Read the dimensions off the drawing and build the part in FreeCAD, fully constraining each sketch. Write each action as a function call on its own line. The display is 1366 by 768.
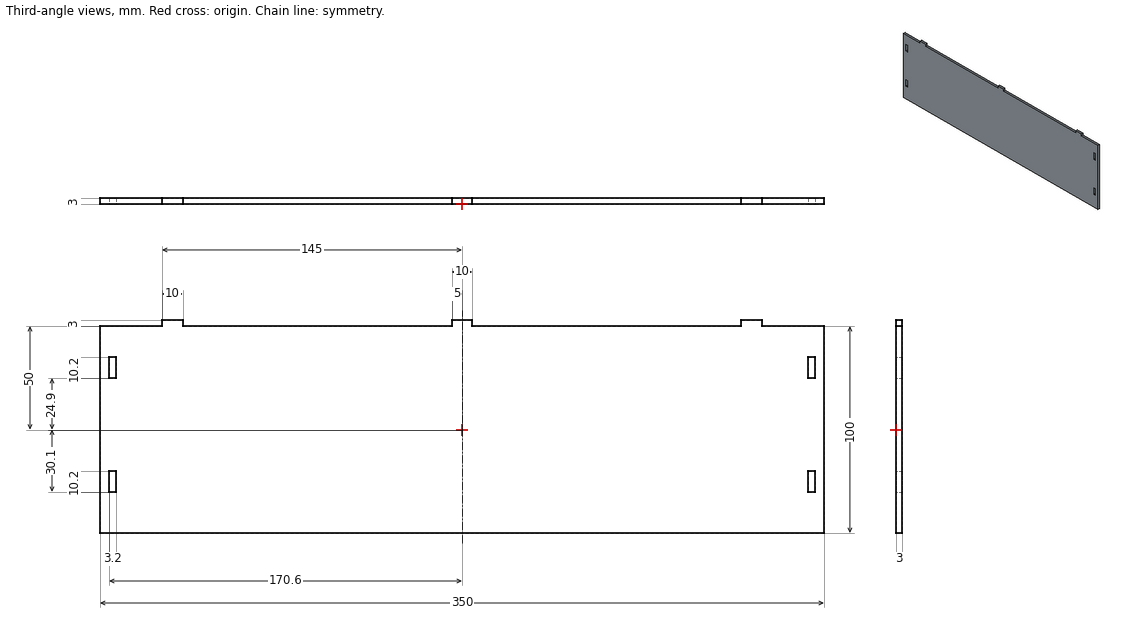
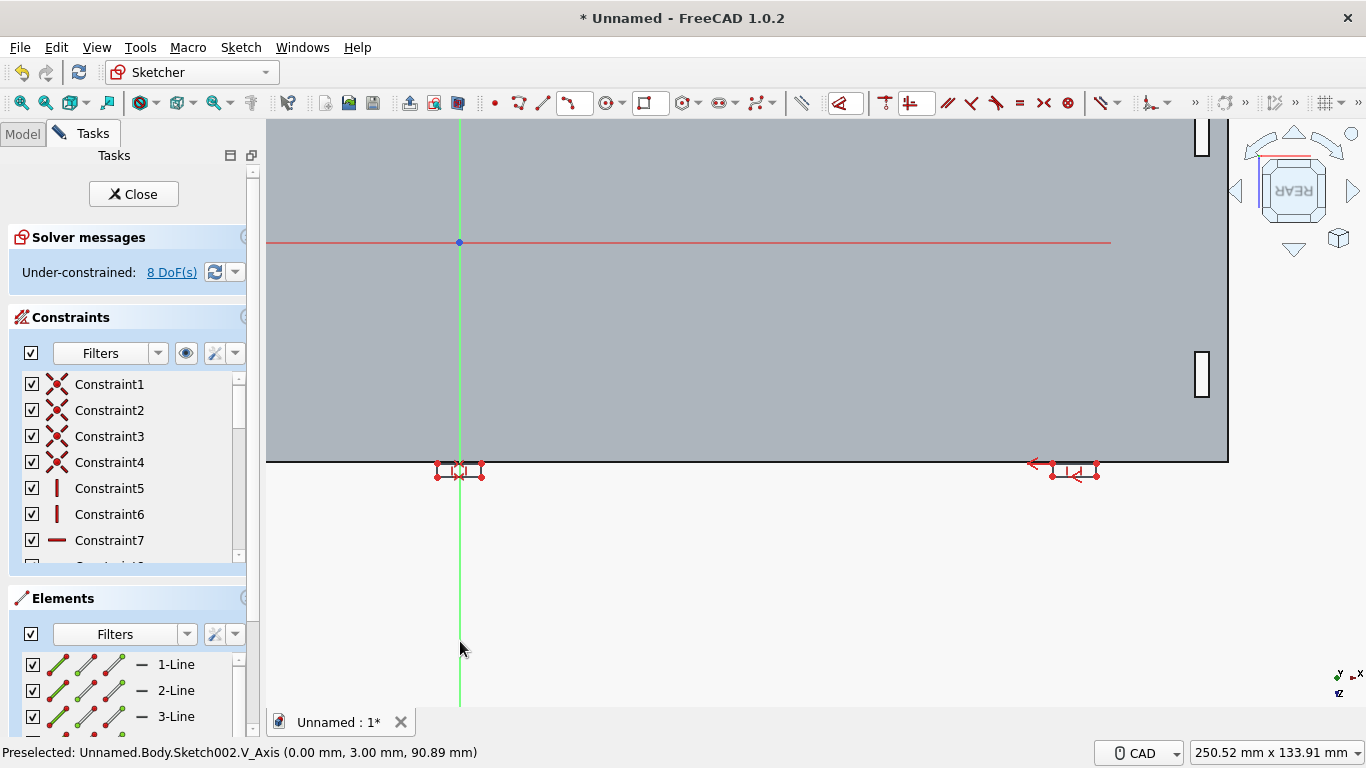
key(d)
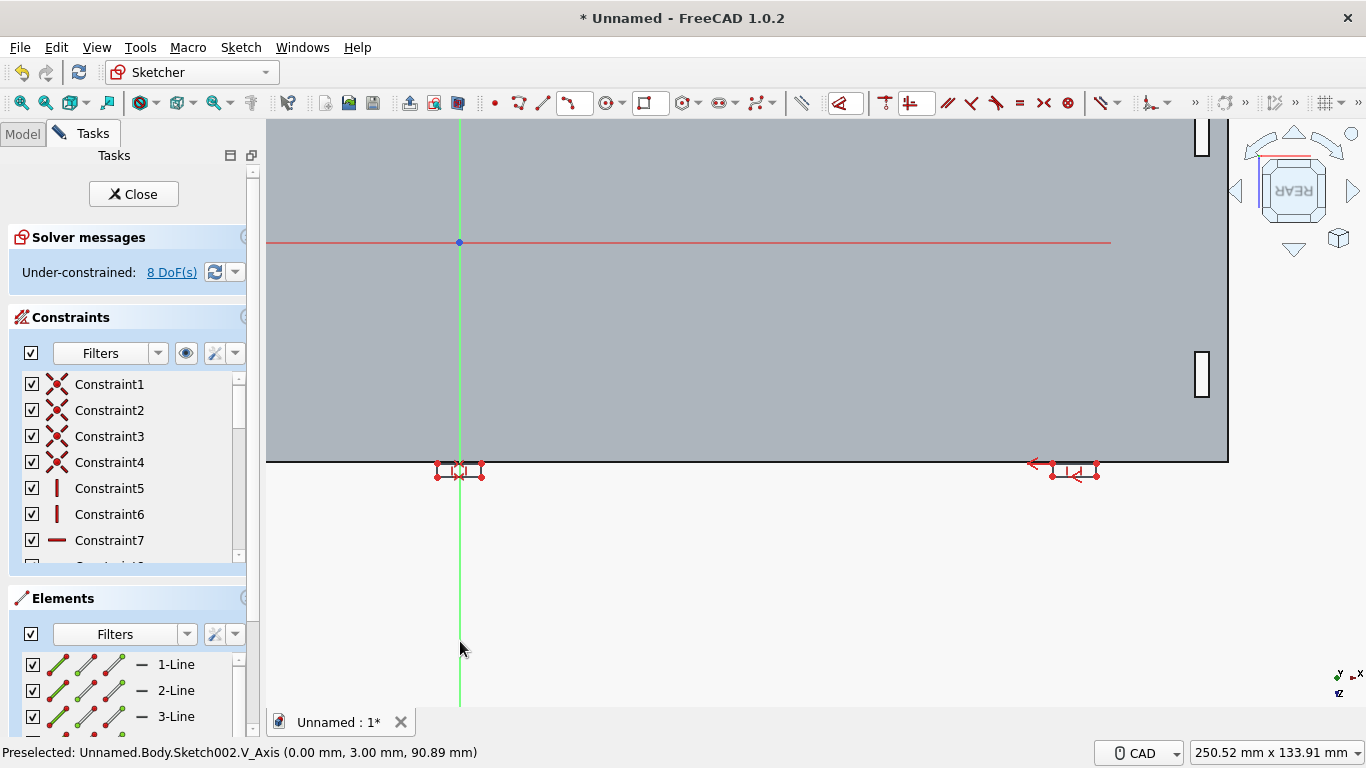
scroll(1097, 478, down, 3)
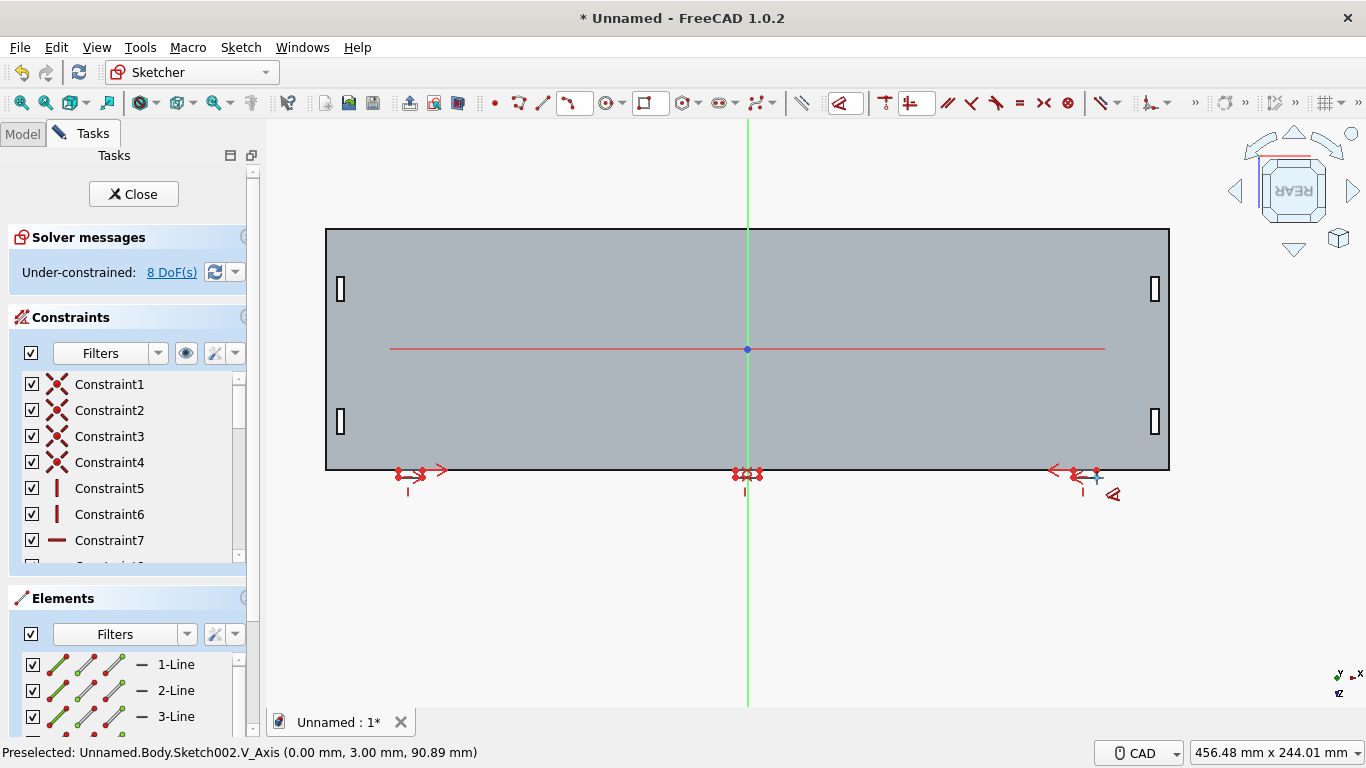
scroll(398, 474, up, 9)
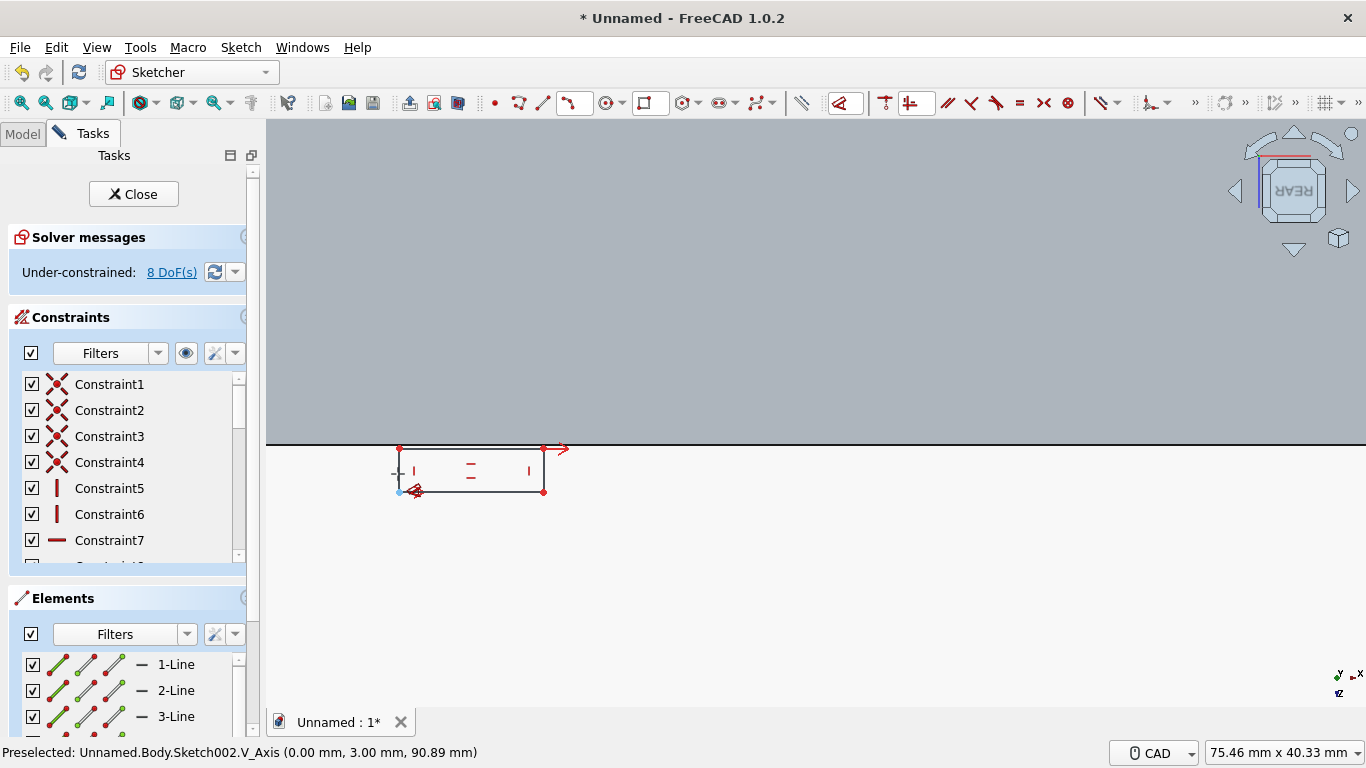
click(399, 470)
click(365, 470)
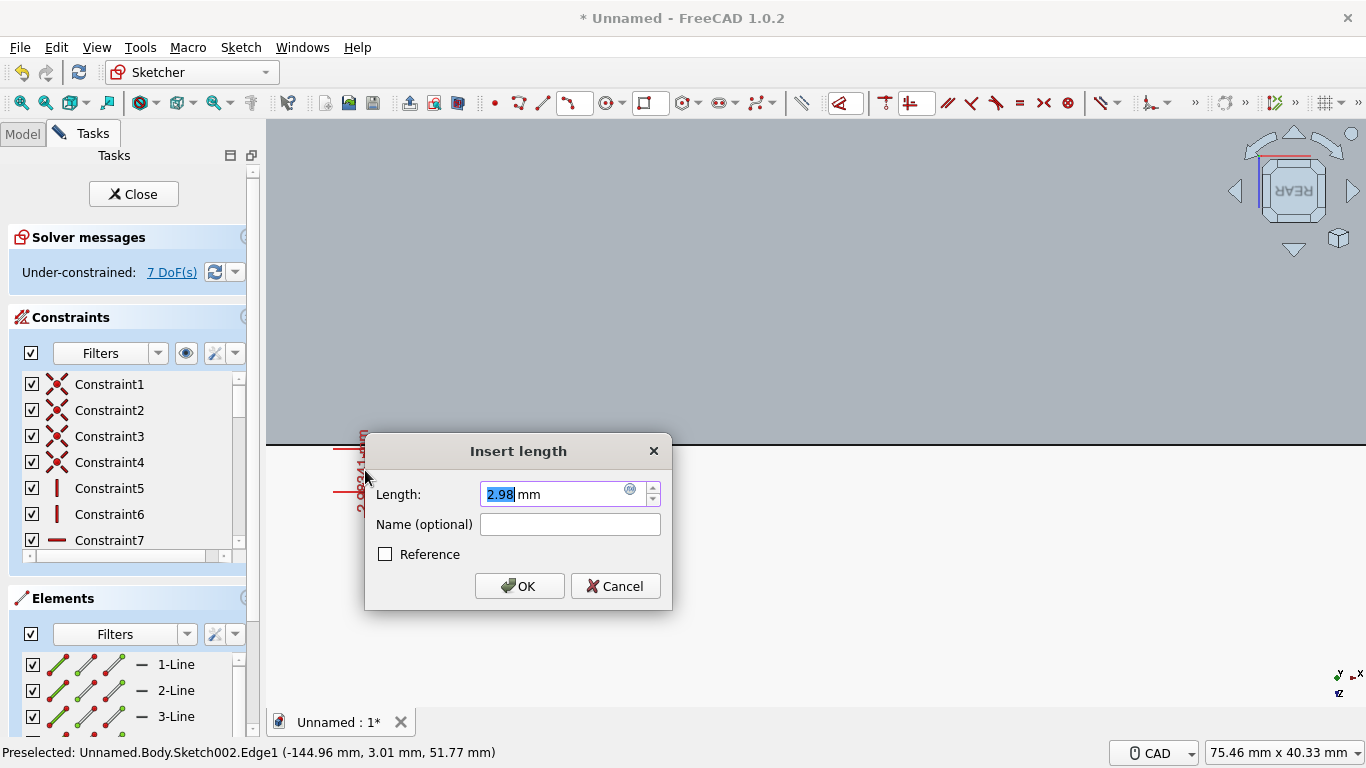
text(3)
key(Return)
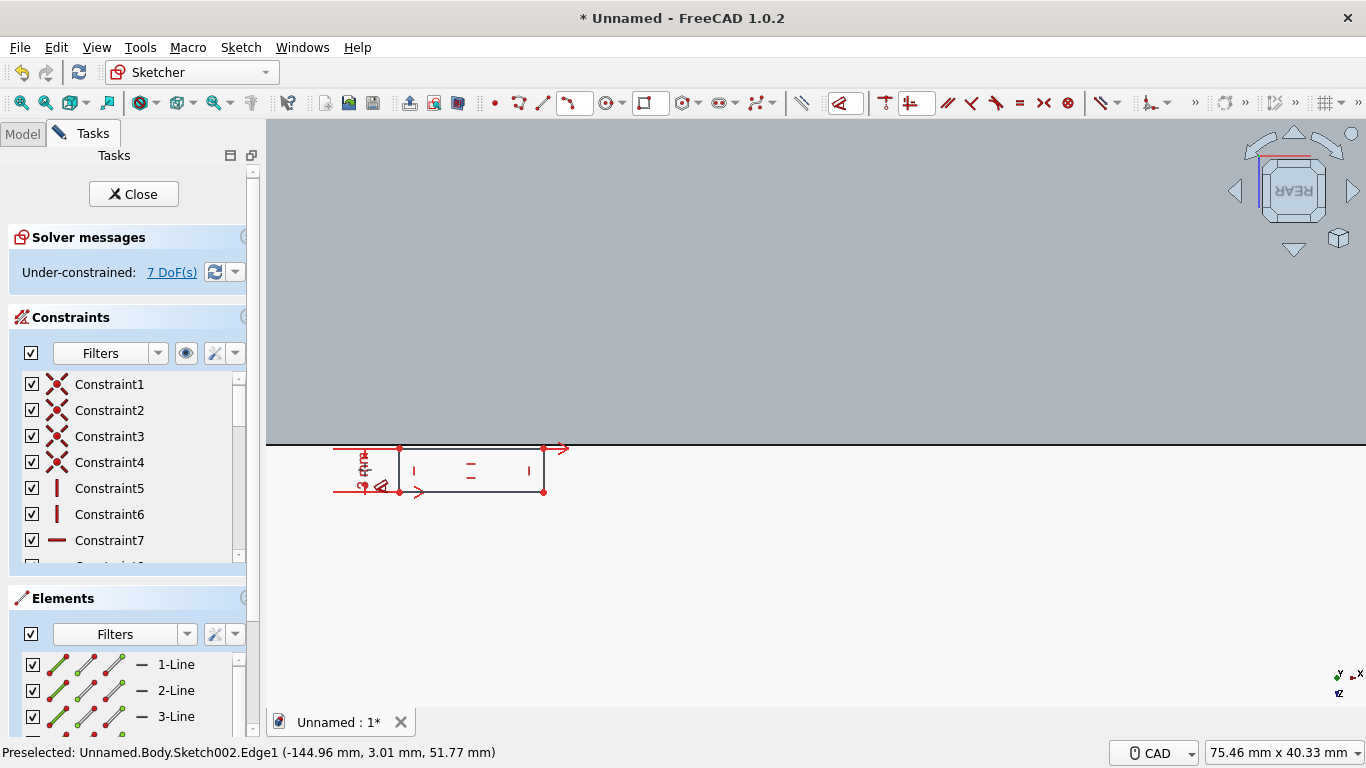
scroll(398, 474, down, 9)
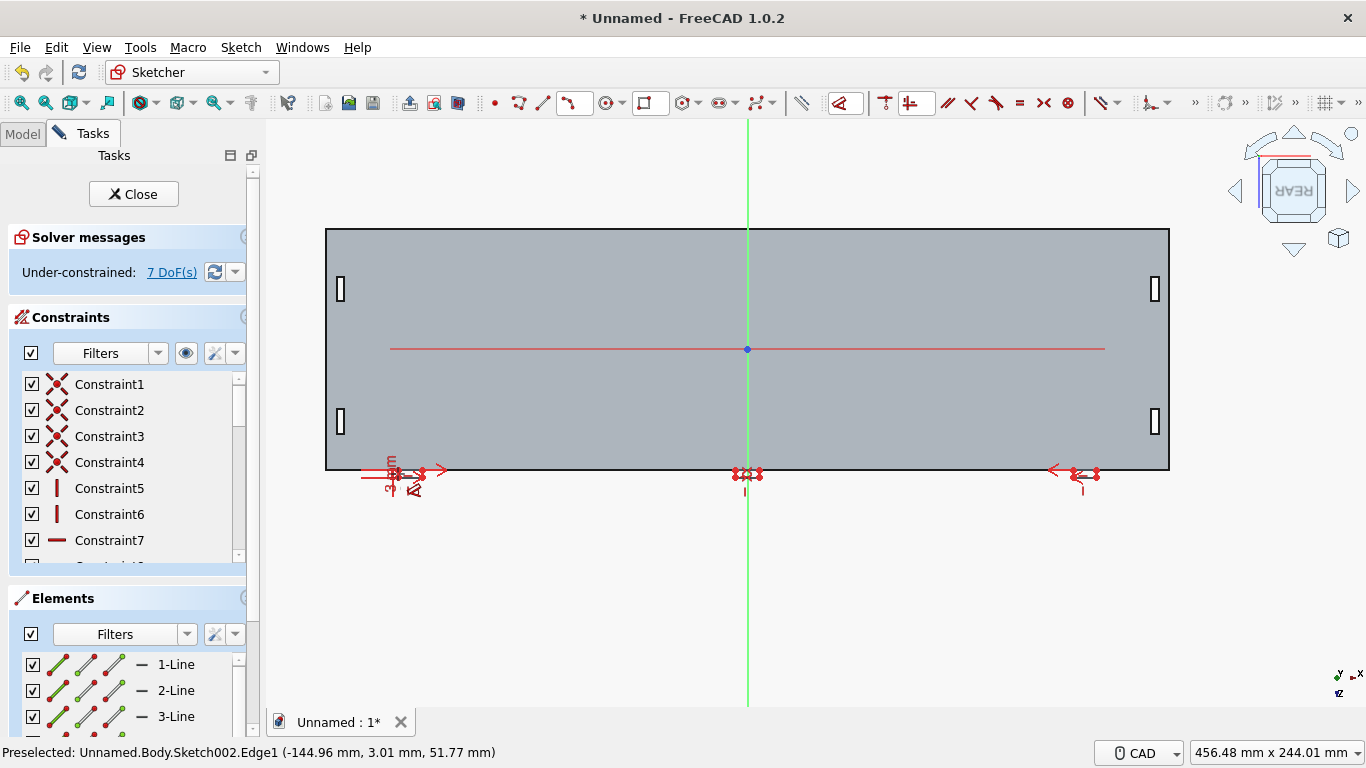
scroll(735, 473, up, 10)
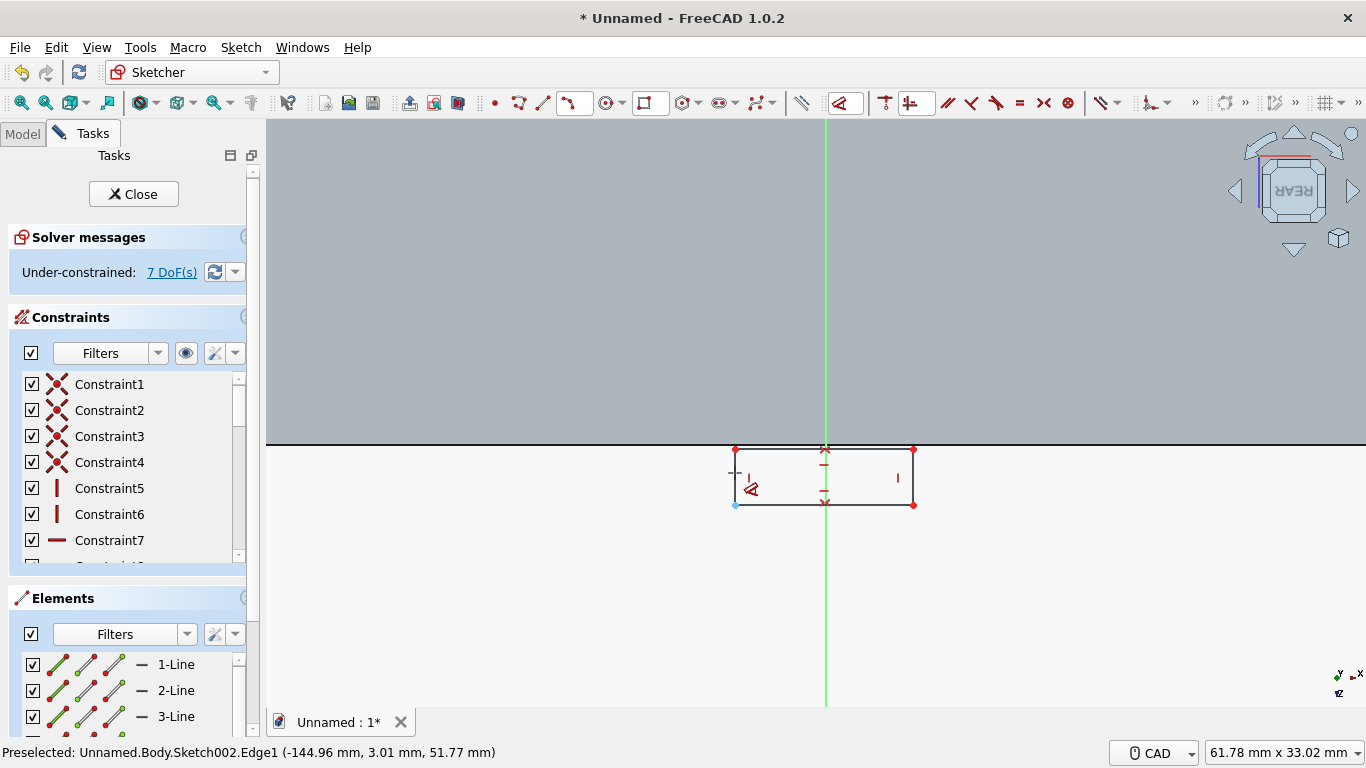
click(735, 466)
click(701, 477)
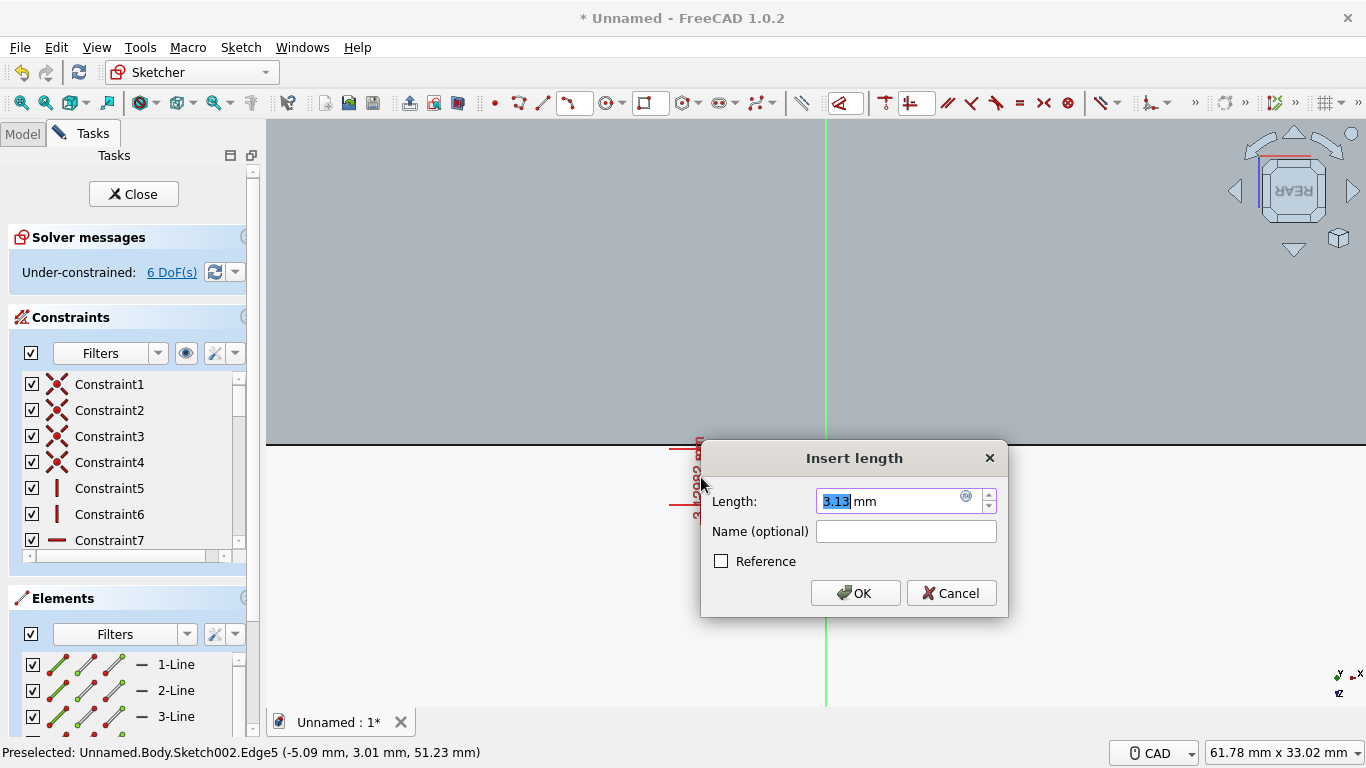
text(3)
key(Return)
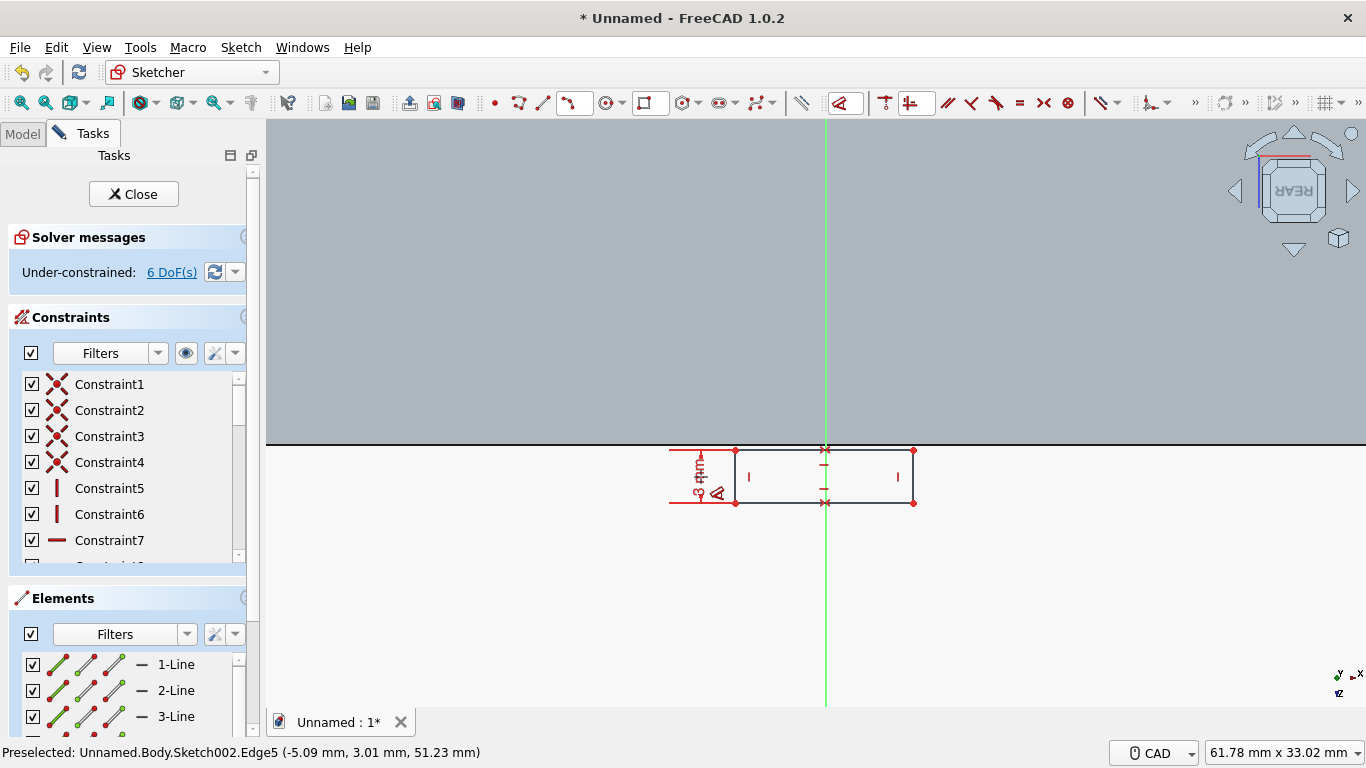
scroll(735, 473, down, 10)